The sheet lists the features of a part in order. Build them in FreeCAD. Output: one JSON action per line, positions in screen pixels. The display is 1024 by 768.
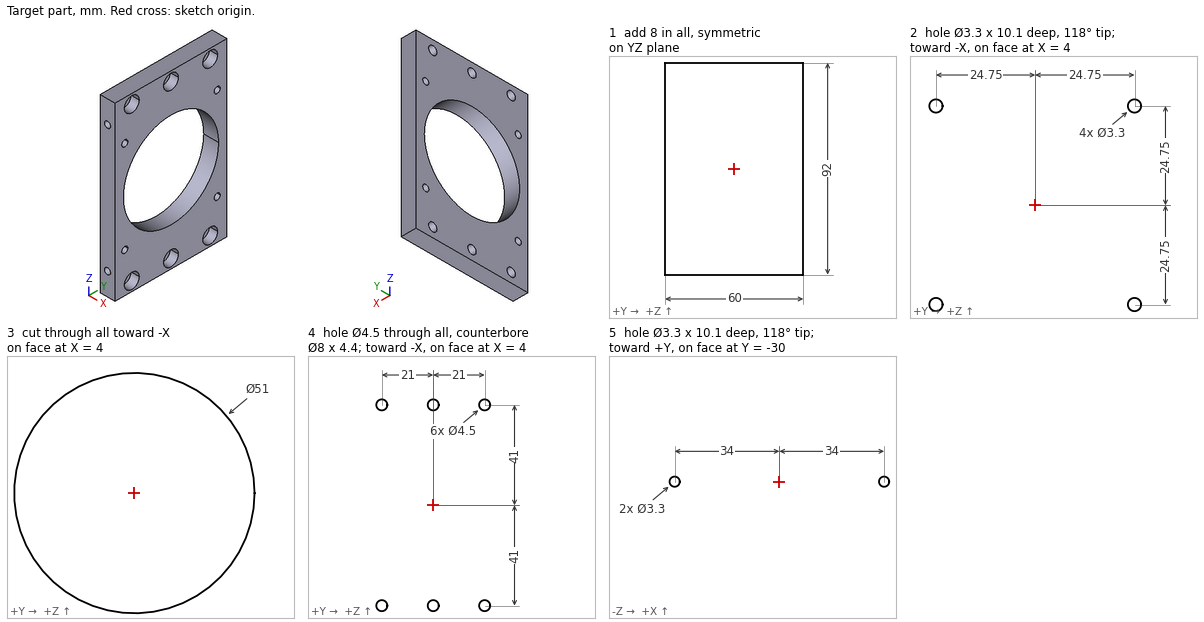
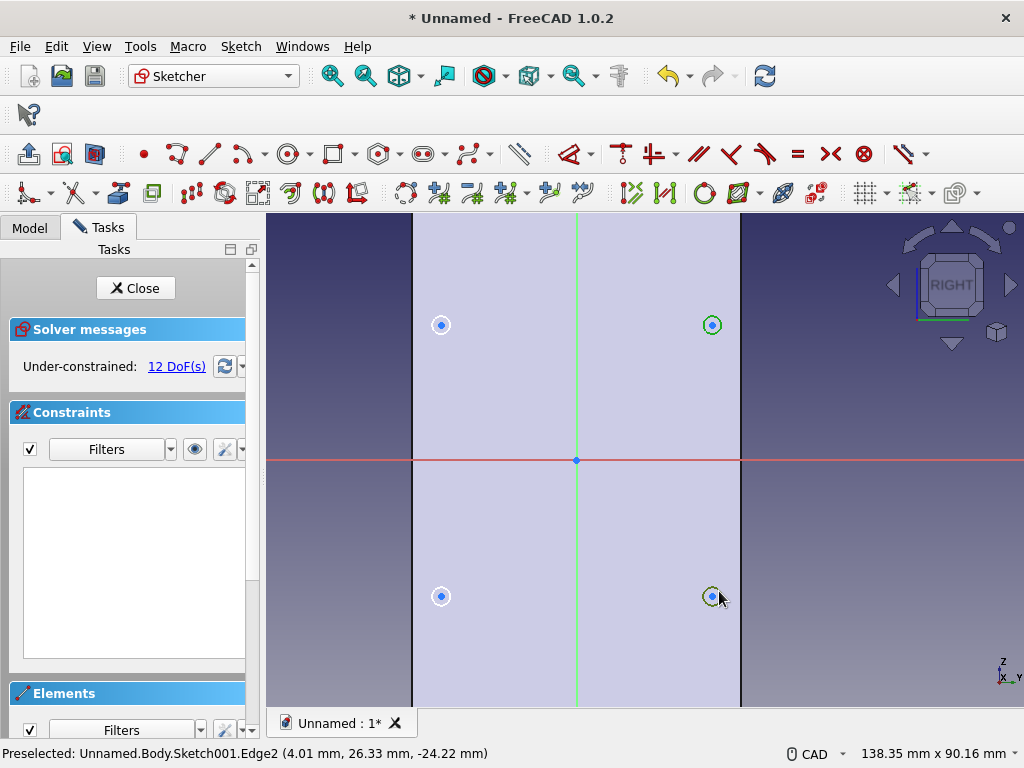
{"action": "scroll", "coordinate": [447, 319], "scroll_direction": "up", "scroll_amount": 3}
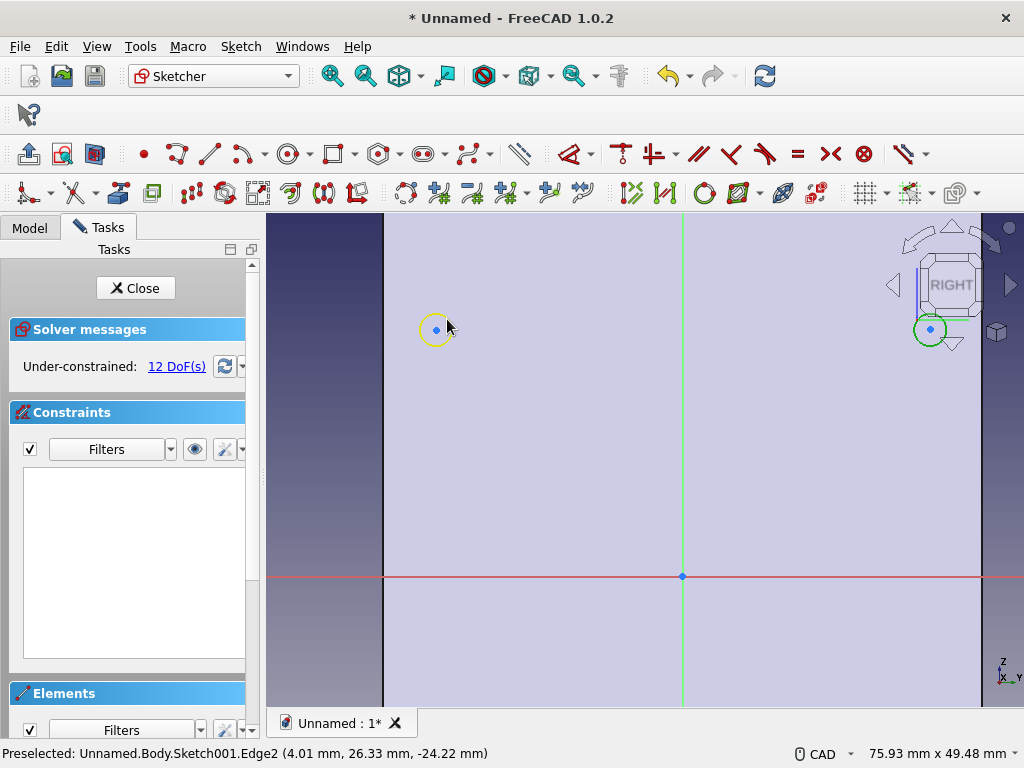
{"action": "left_click", "coordinate": [447, 319]}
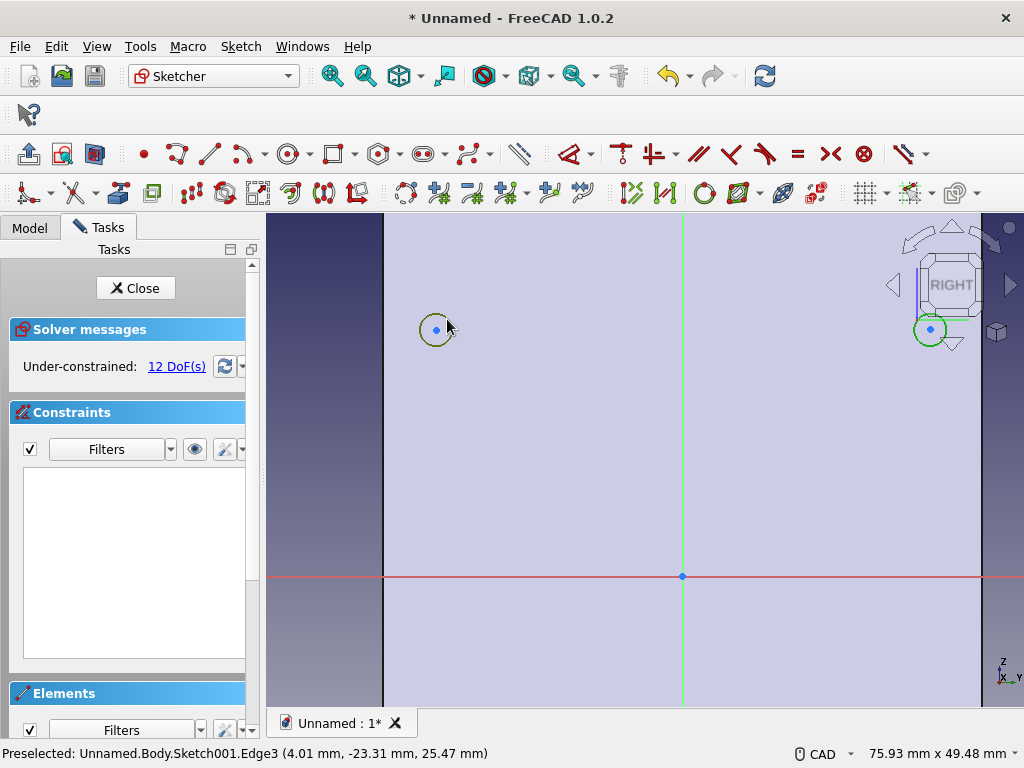
{"action": "scroll", "coordinate": [447, 318], "scroll_direction": "down", "scroll_amount": 3}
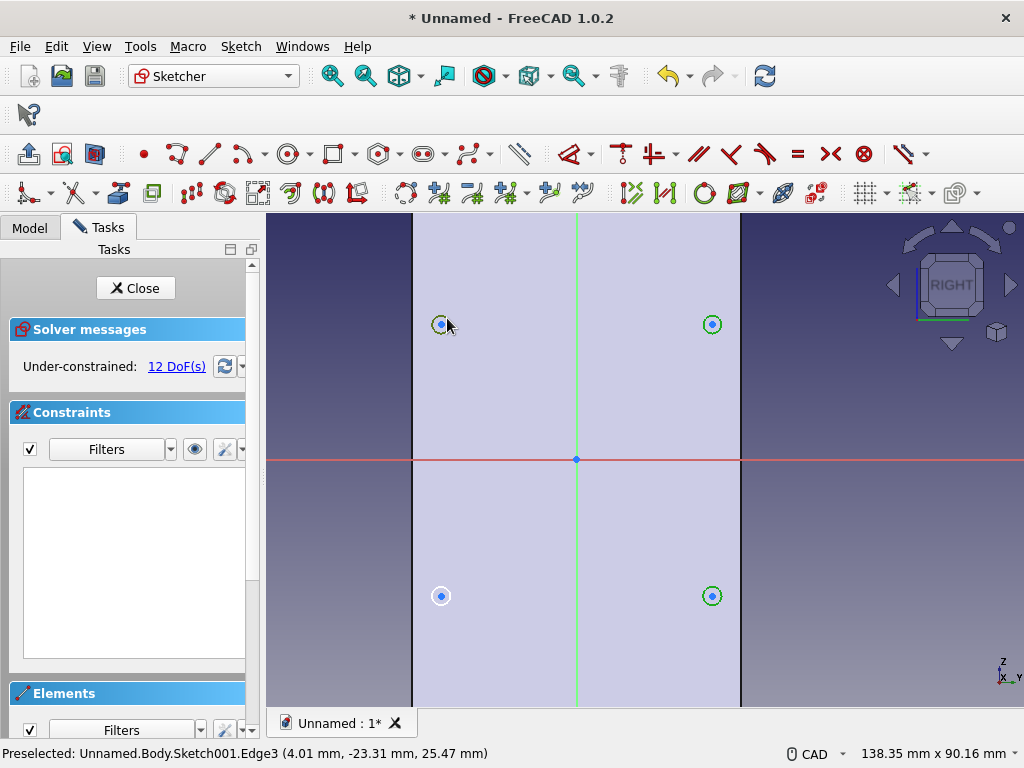
{"action": "scroll", "coordinate": [448, 590], "scroll_direction": "up", "scroll_amount": 3}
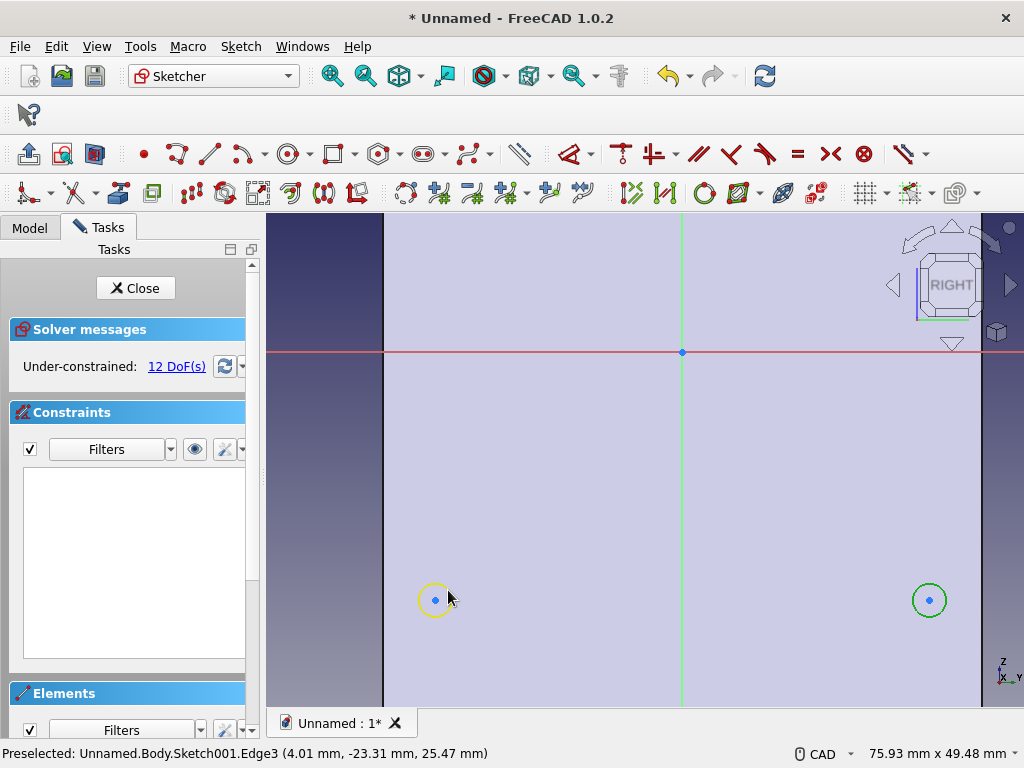
{"action": "left_click", "coordinate": [447, 589]}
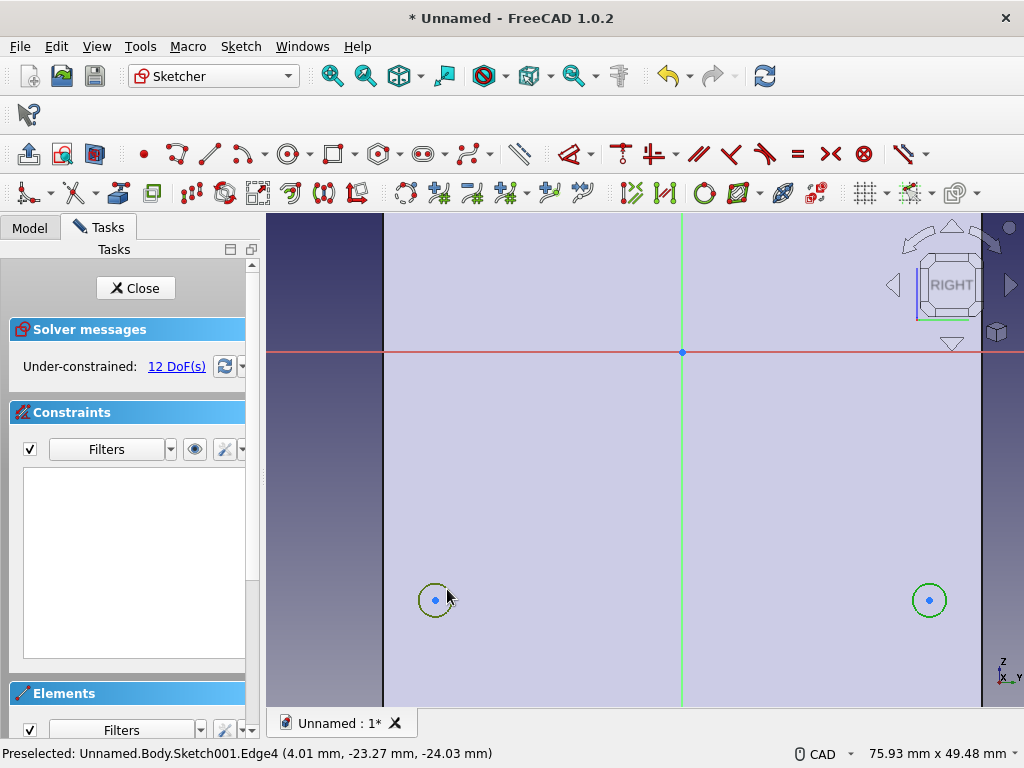
{"action": "left_click", "coordinate": [798, 154]}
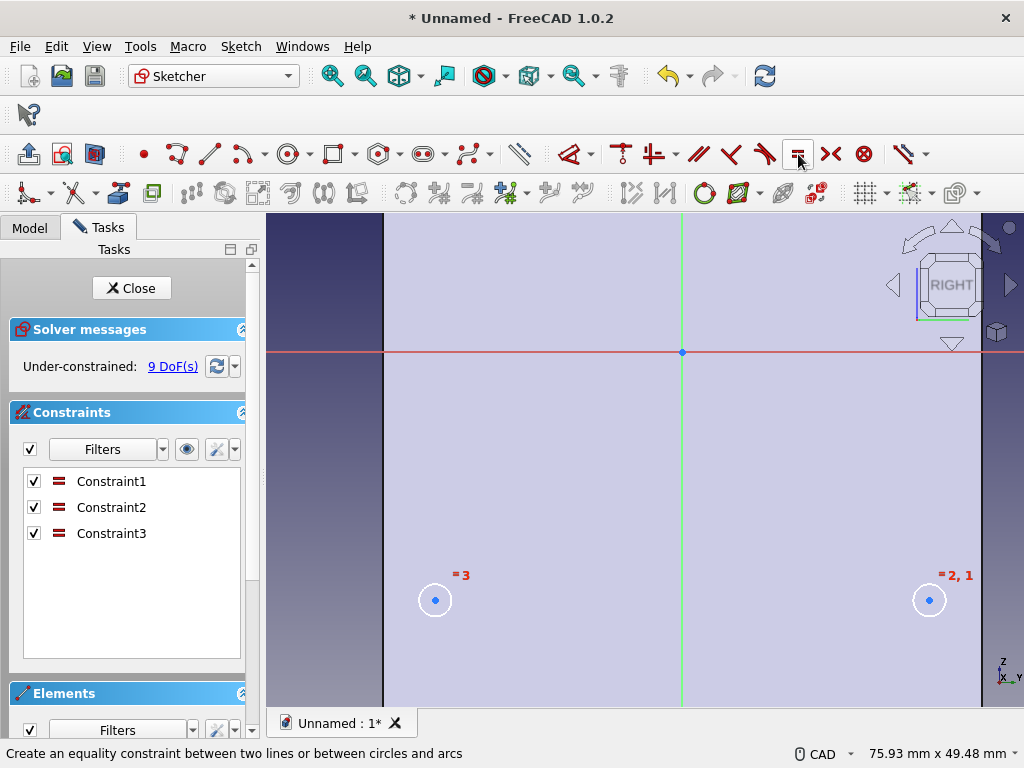
{"action": "scroll", "coordinate": [448, 591], "scroll_direction": "down", "scroll_amount": 3}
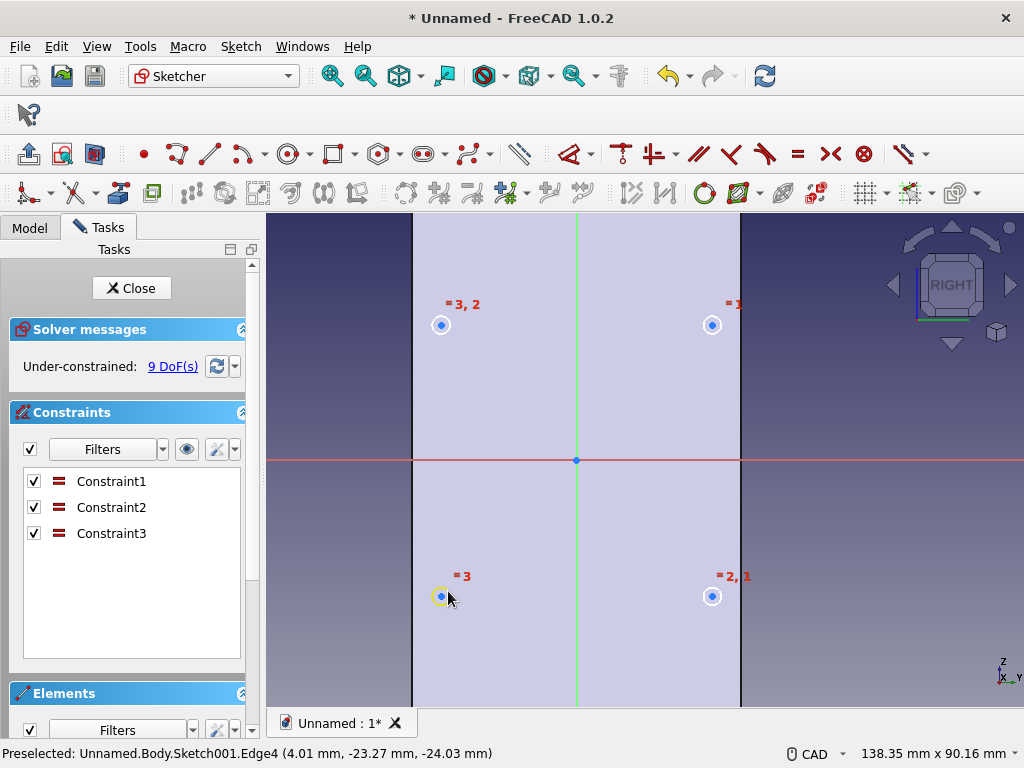
{"action": "left_click", "coordinate": [712, 325]}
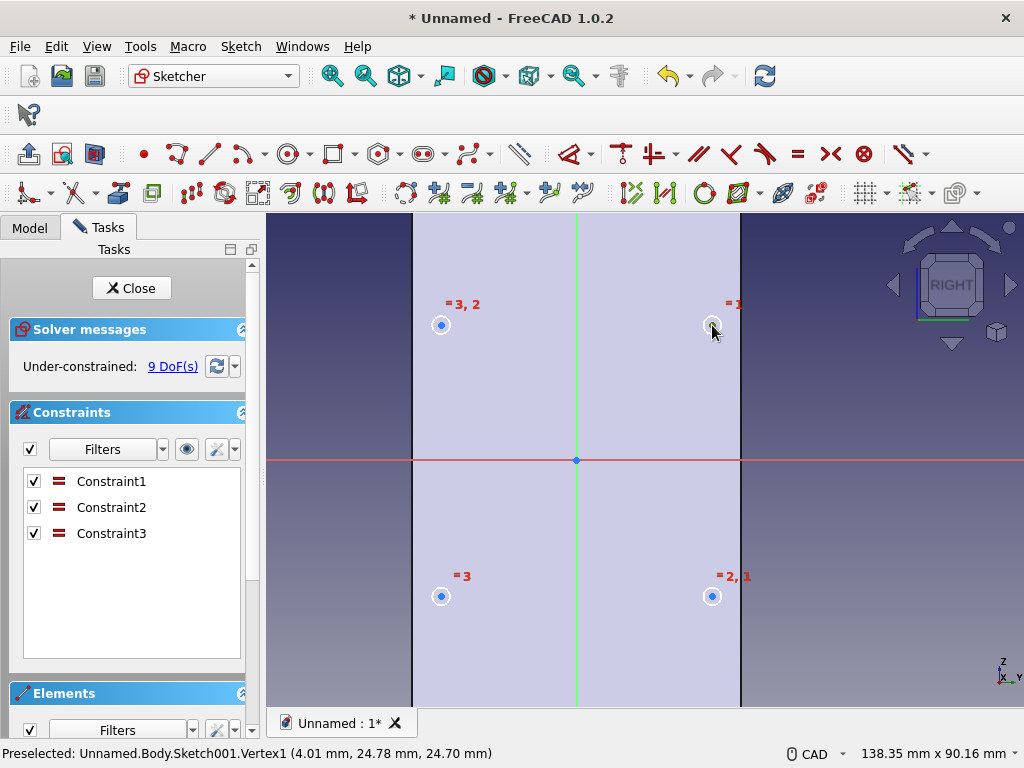
{"action": "left_click", "coordinate": [712, 596]}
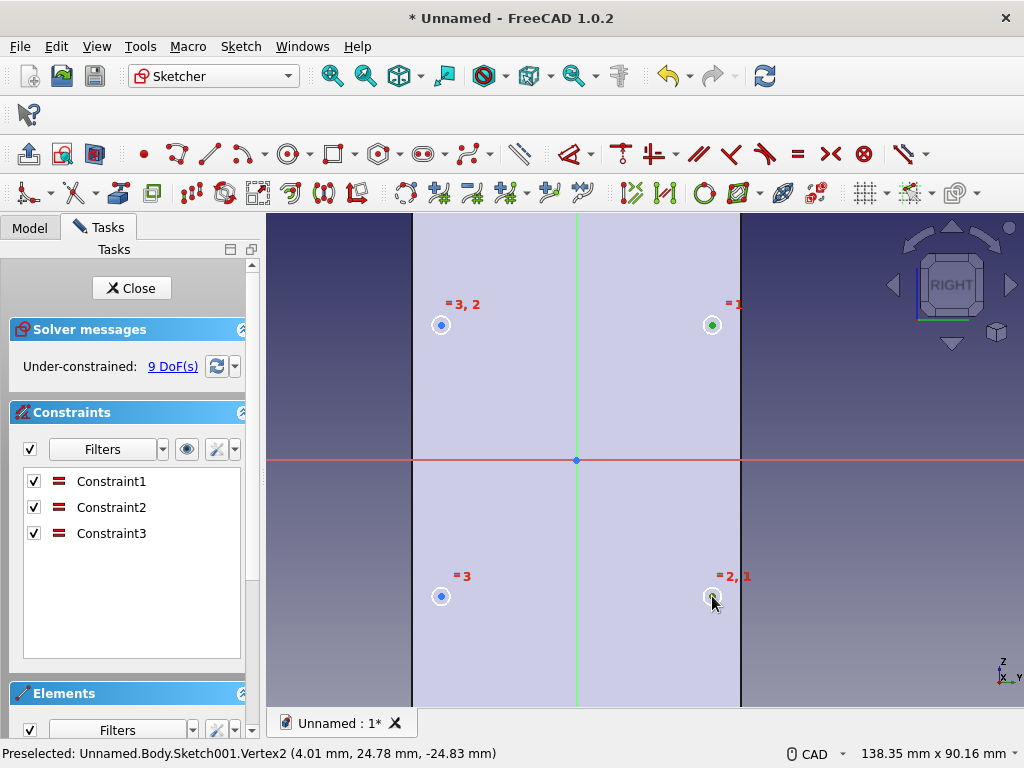
{"action": "left_click", "coordinate": [676, 154]}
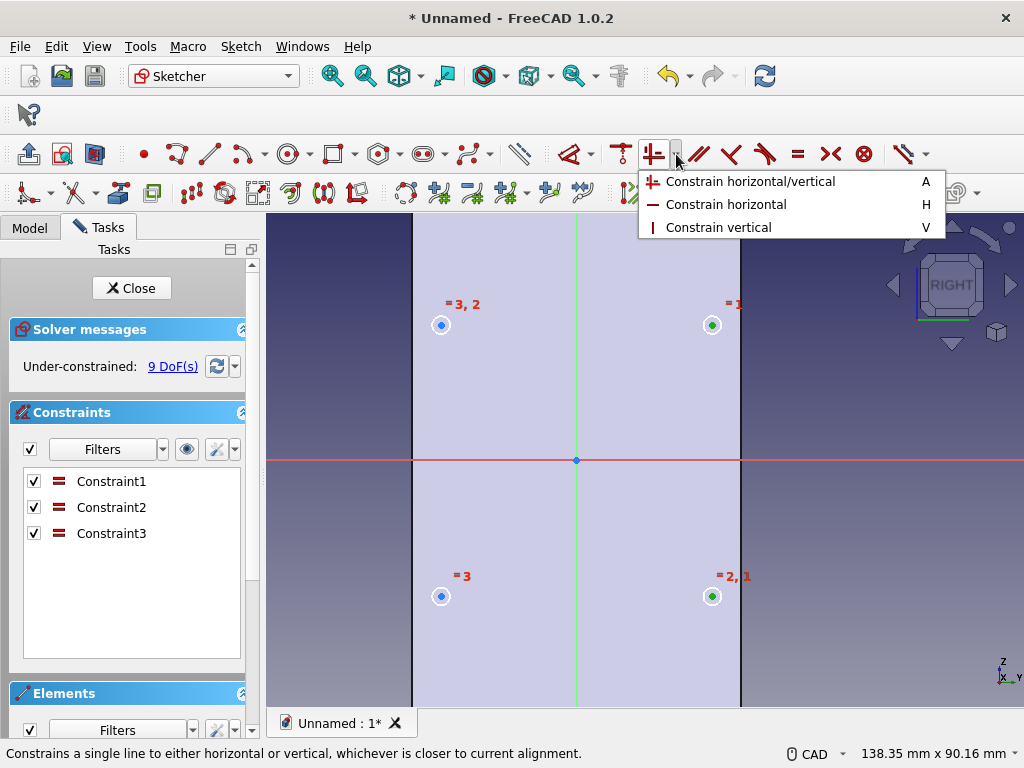
{"action": "left_click", "coordinate": [792, 228]}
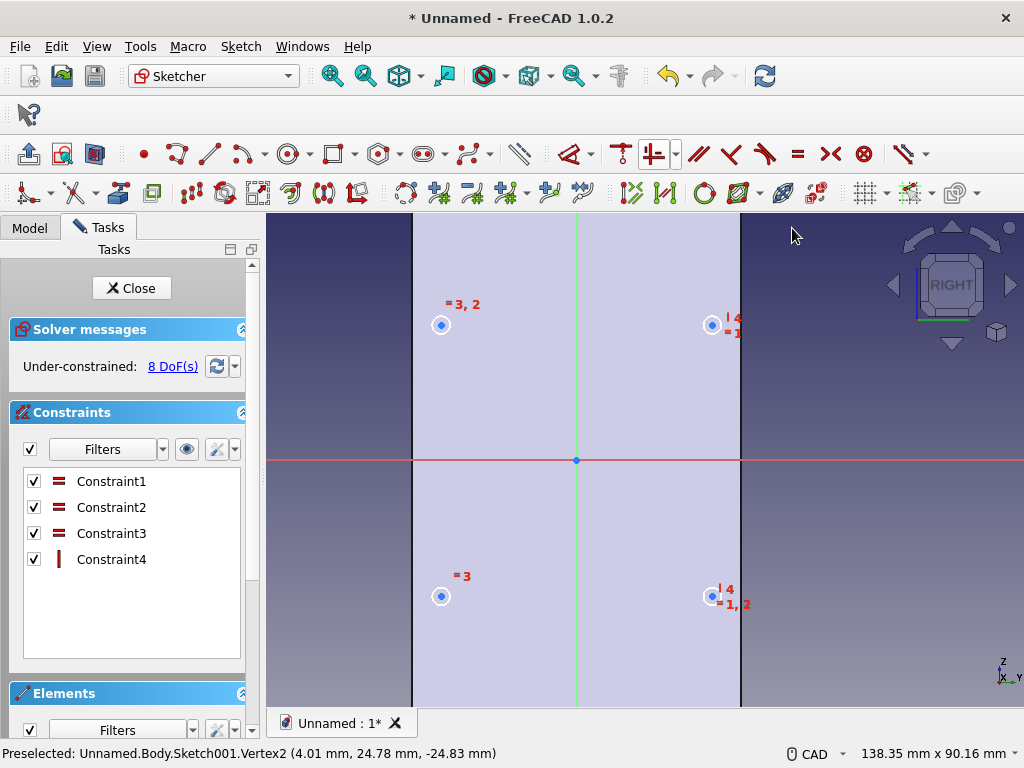
{"action": "left_click", "coordinate": [712, 325]}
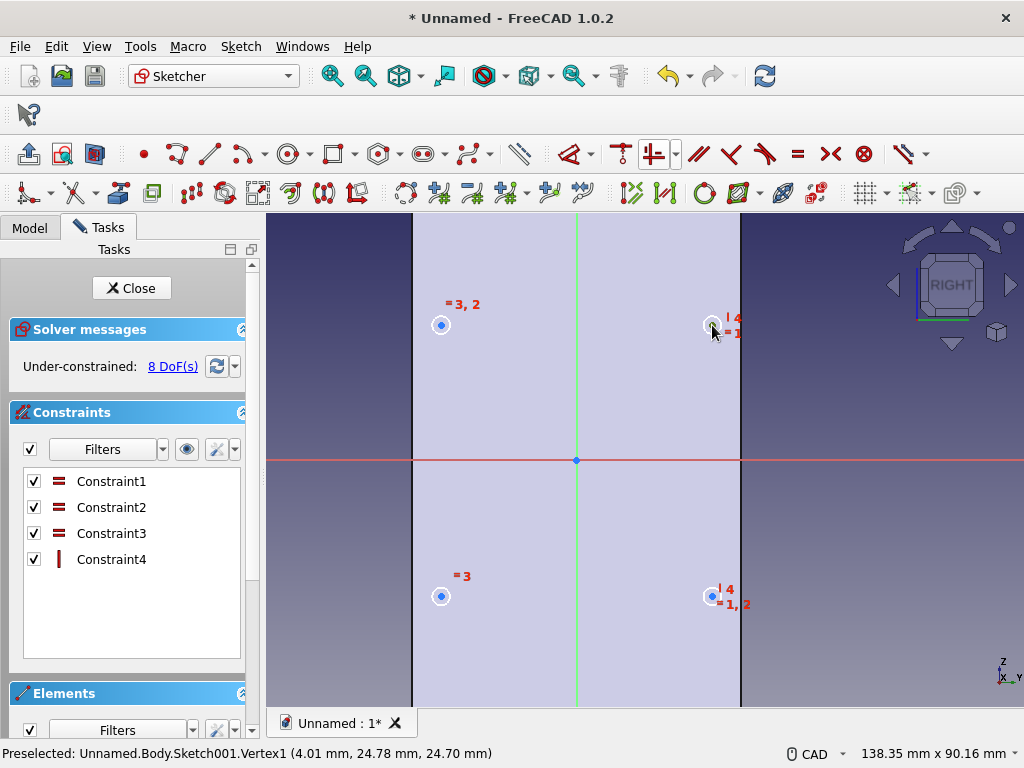
{"action": "left_click", "coordinate": [441, 325]}